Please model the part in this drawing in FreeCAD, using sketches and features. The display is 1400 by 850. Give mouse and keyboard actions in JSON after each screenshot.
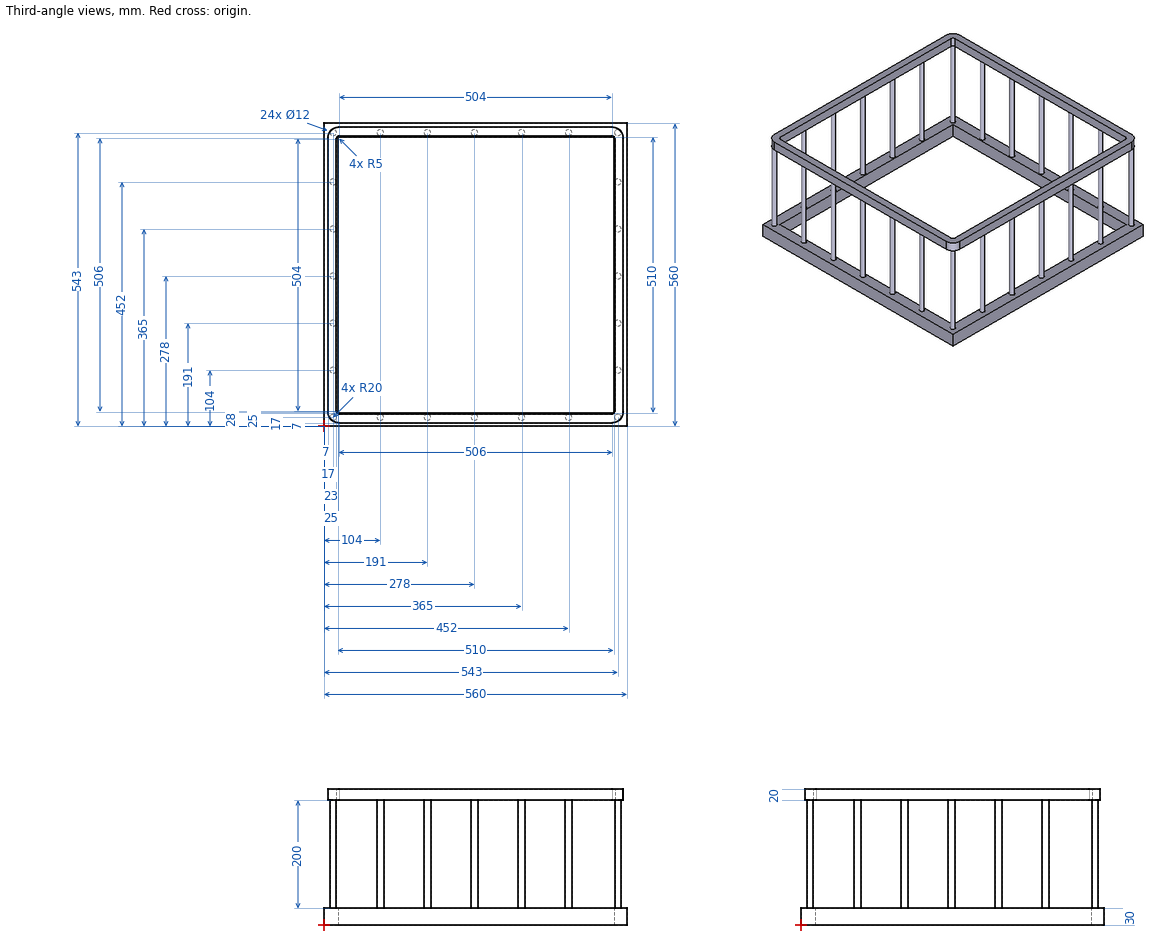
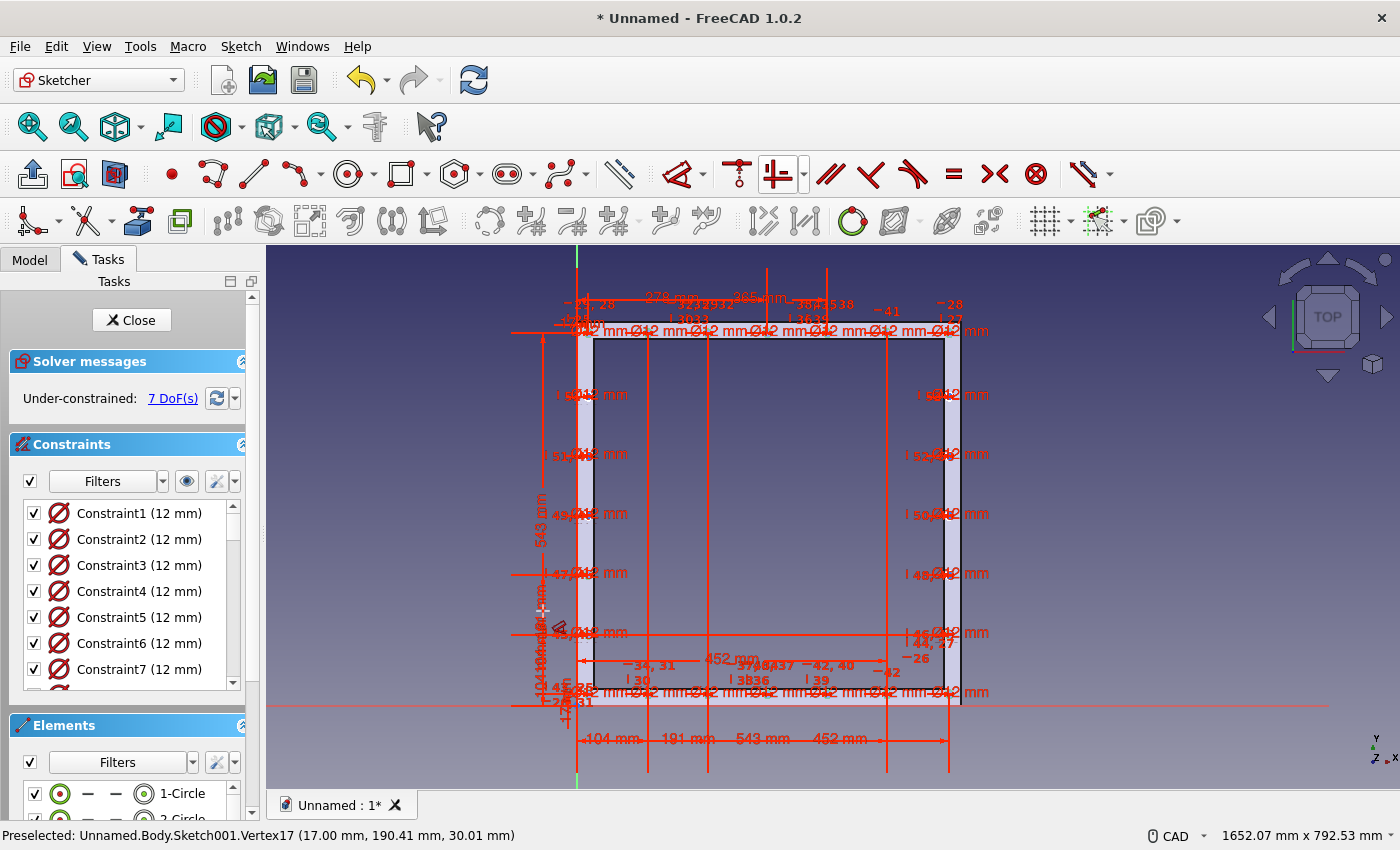
{"action": "left_click", "coordinate": [949, 575]}
{"action": "left_click", "coordinate": [983, 641]}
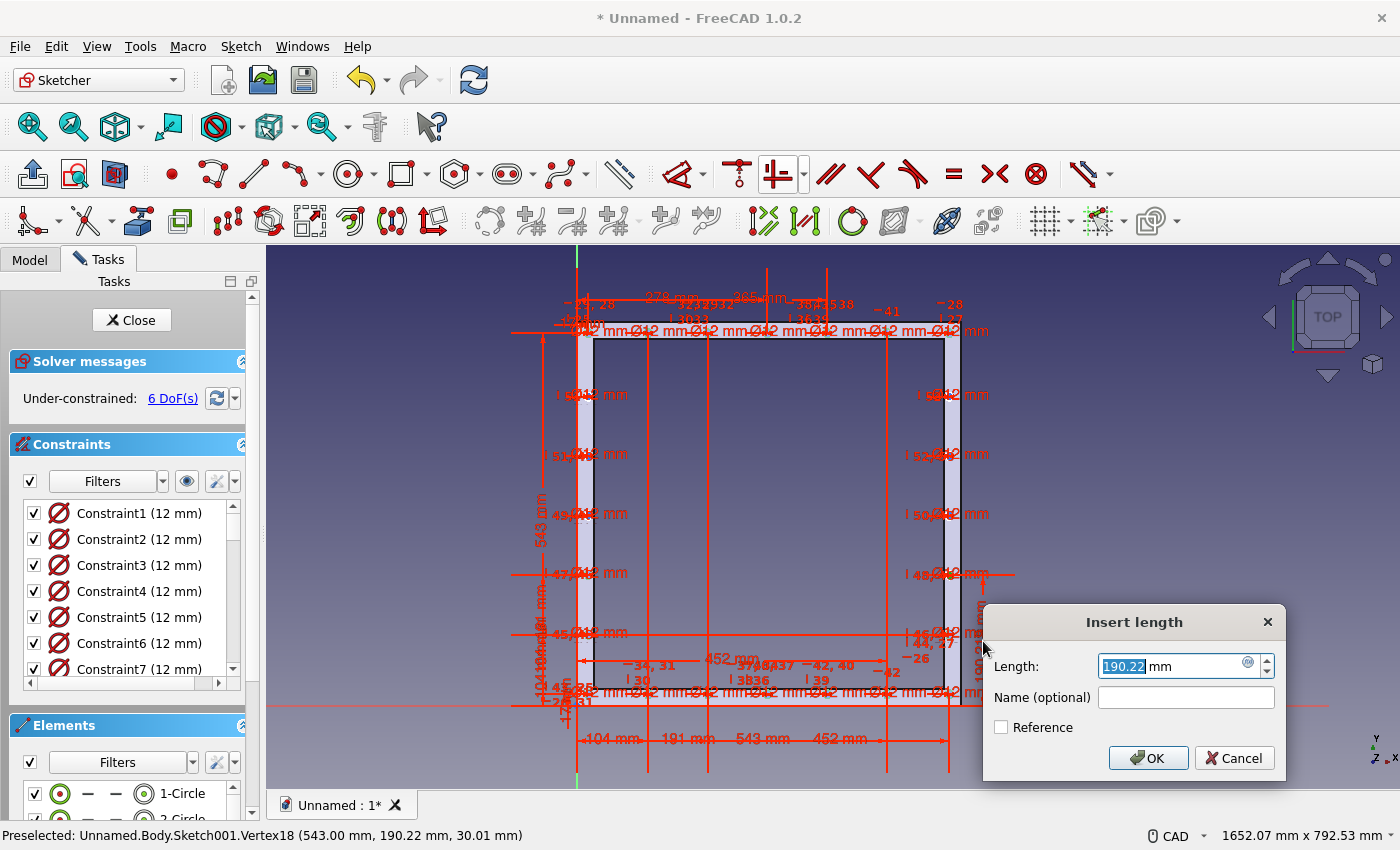
{"action": "type", "text": "191"}
{"action": "key", "text": "Return"}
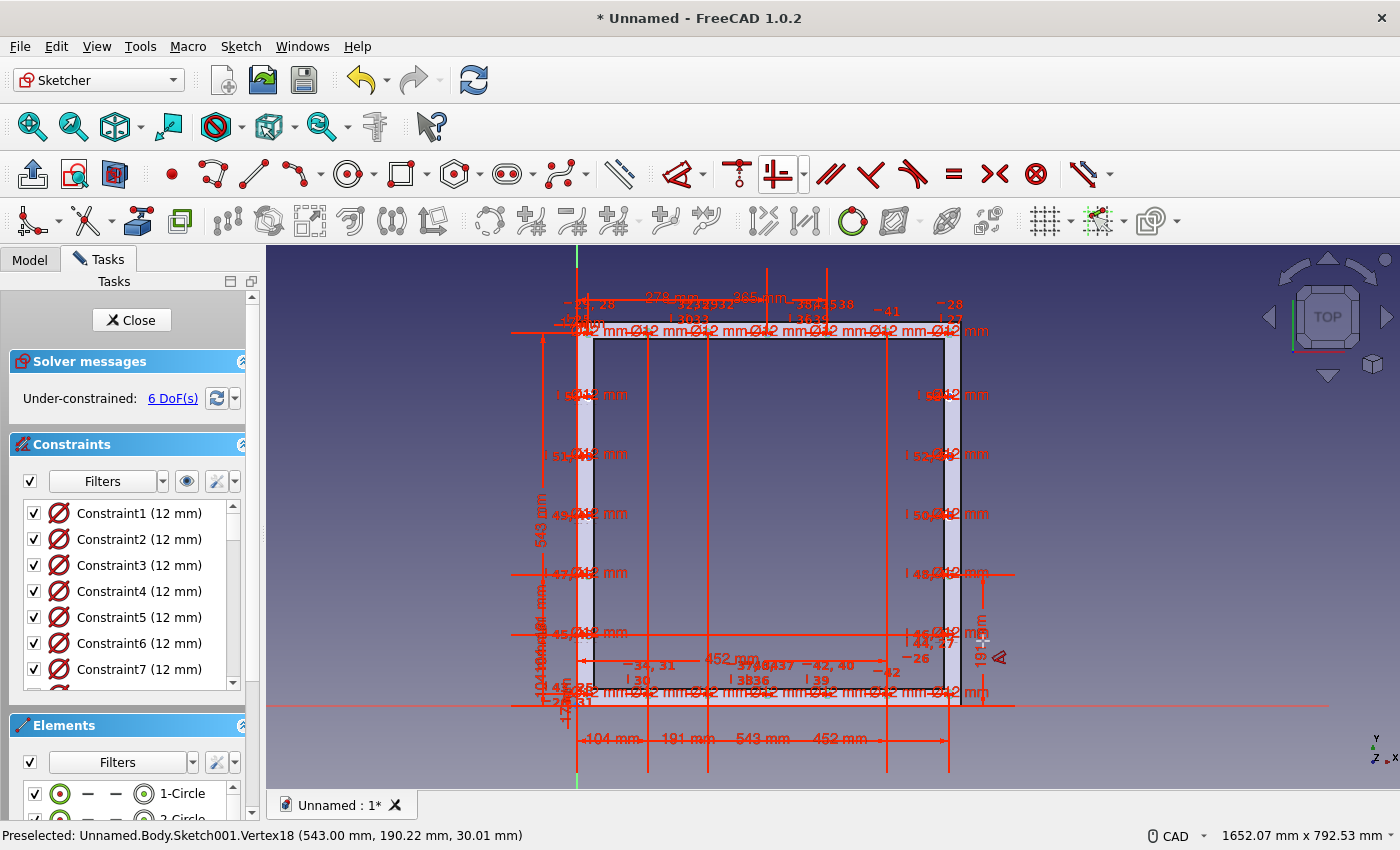
{"action": "left_click", "coordinate": [588, 516]}
{"action": "left_click", "coordinate": [543, 567]}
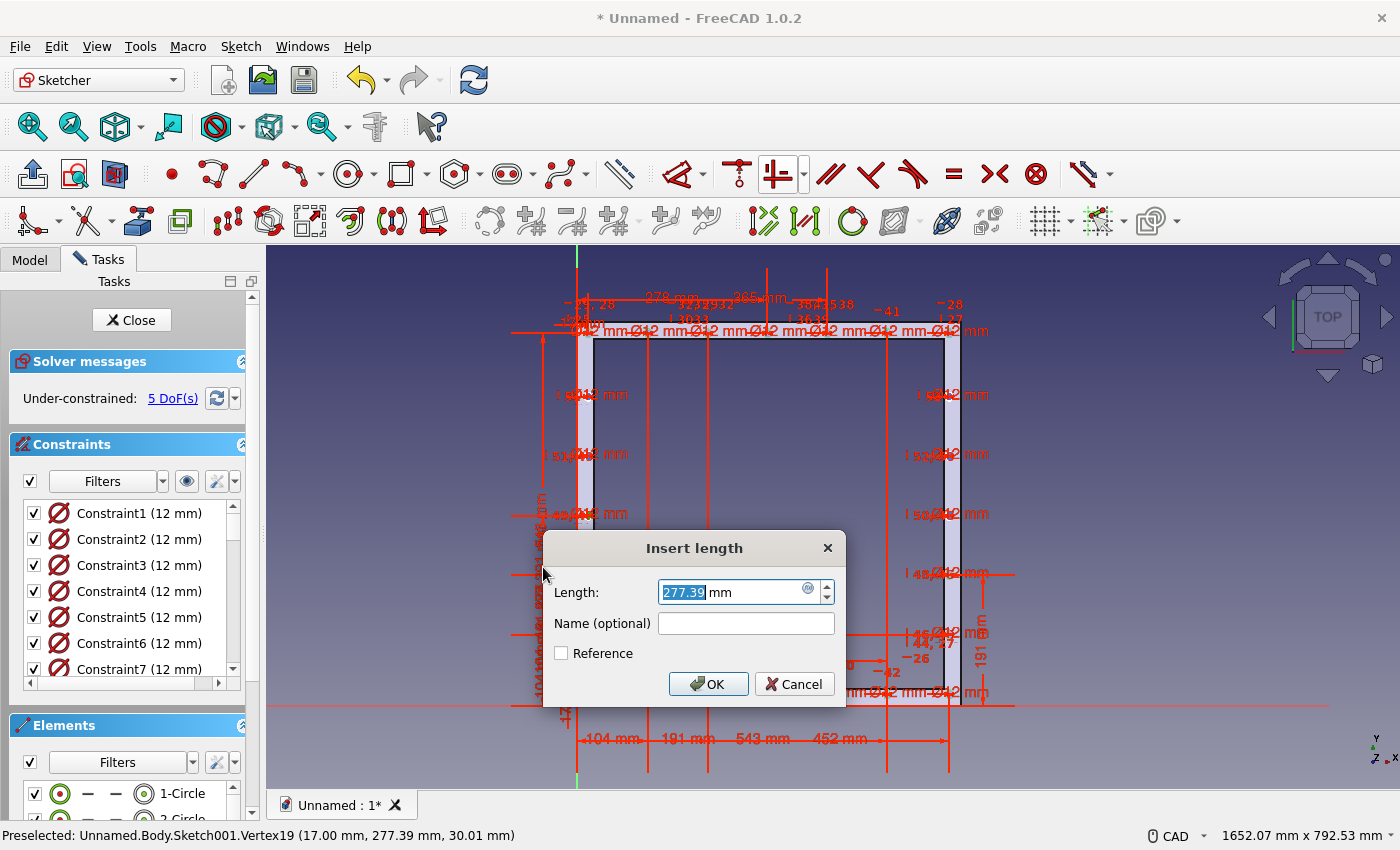
{"action": "type", "text": "278"}
{"action": "key", "text": "Return"}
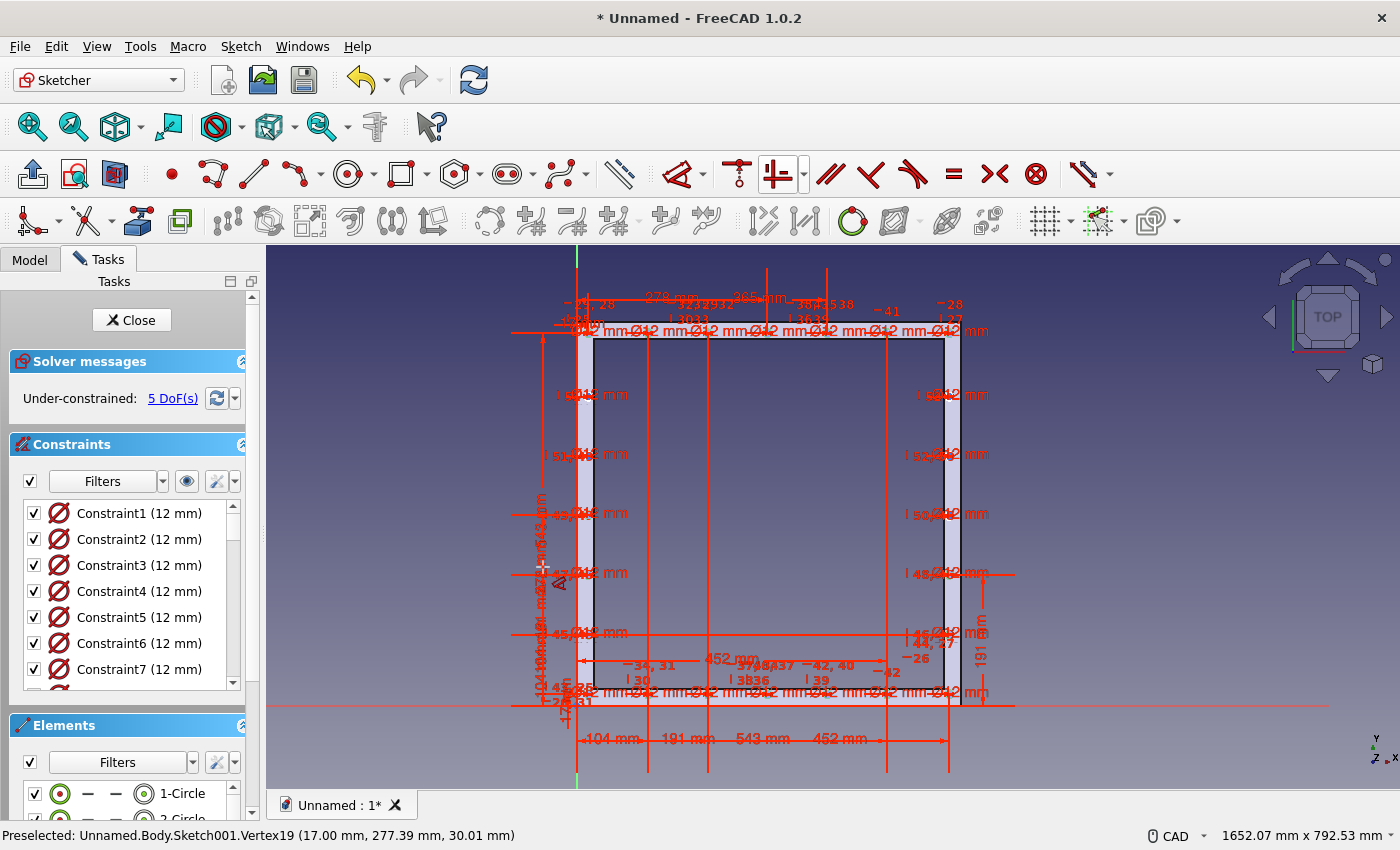
{"action": "left_click", "coordinate": [949, 516]}
{"action": "left_click", "coordinate": [543, 544]}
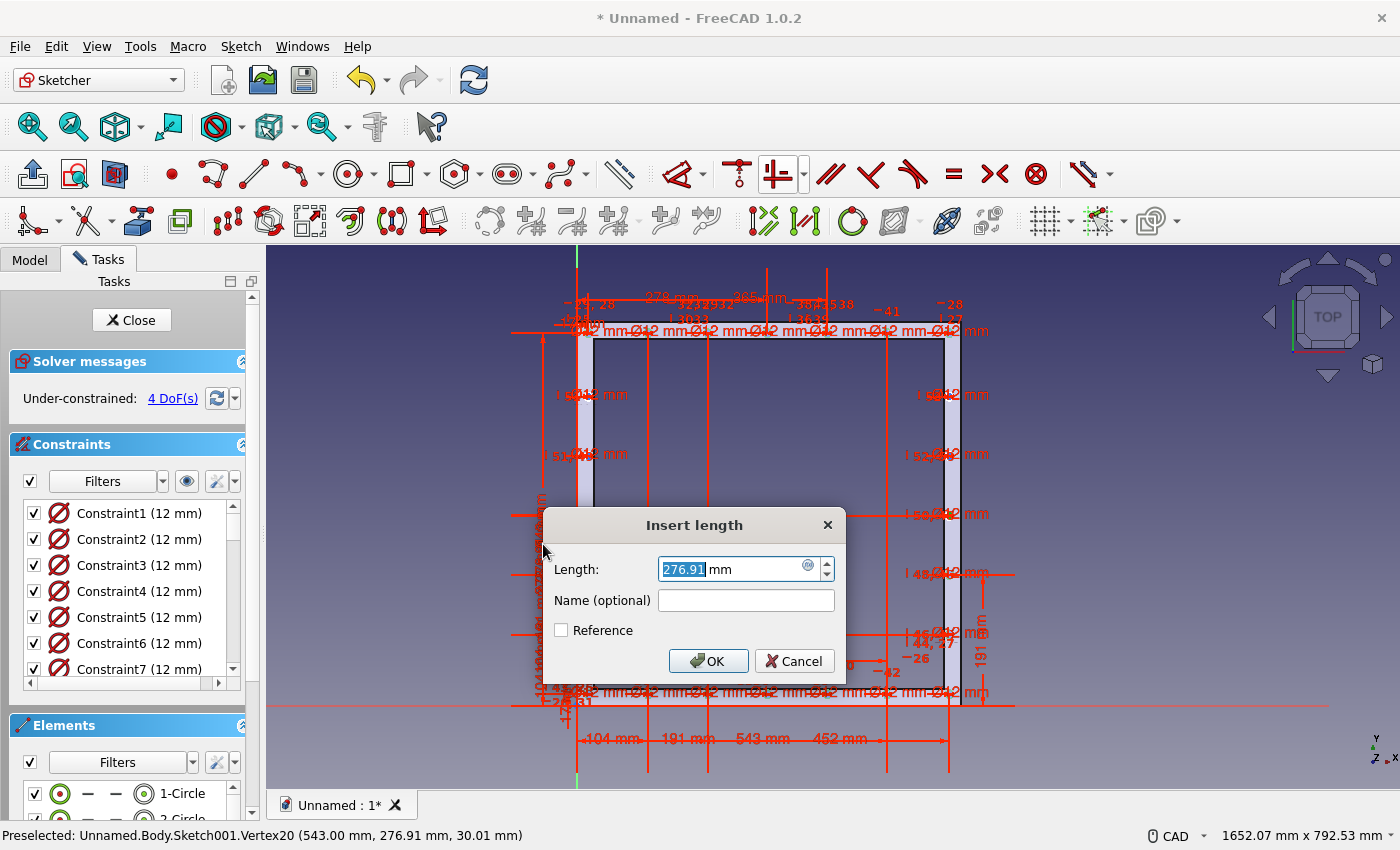
{"action": "type", "text": "278"}
{"action": "key", "text": "Return"}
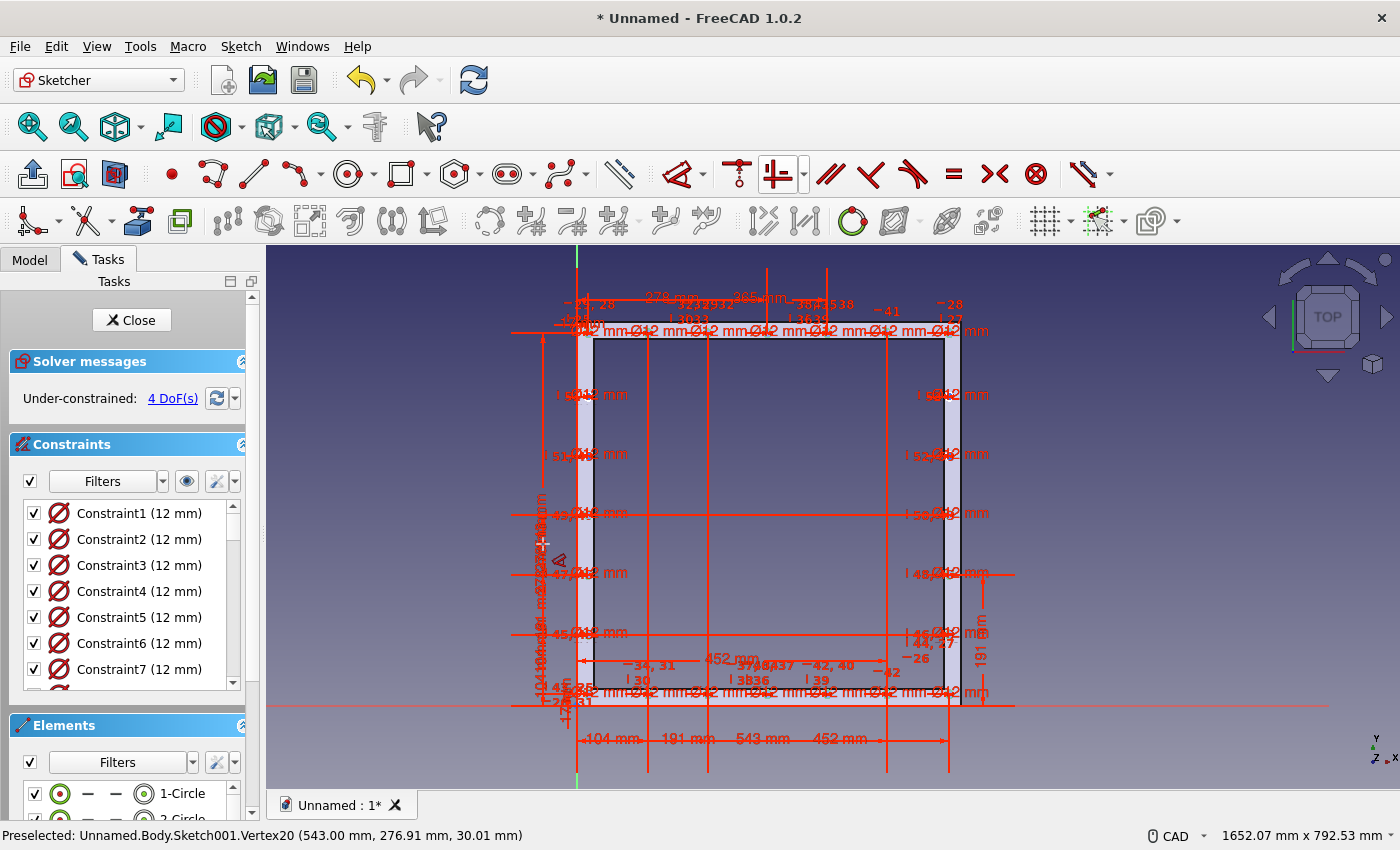
{"action": "left_click", "coordinate": [588, 456]}
{"action": "left_click", "coordinate": [543, 494]}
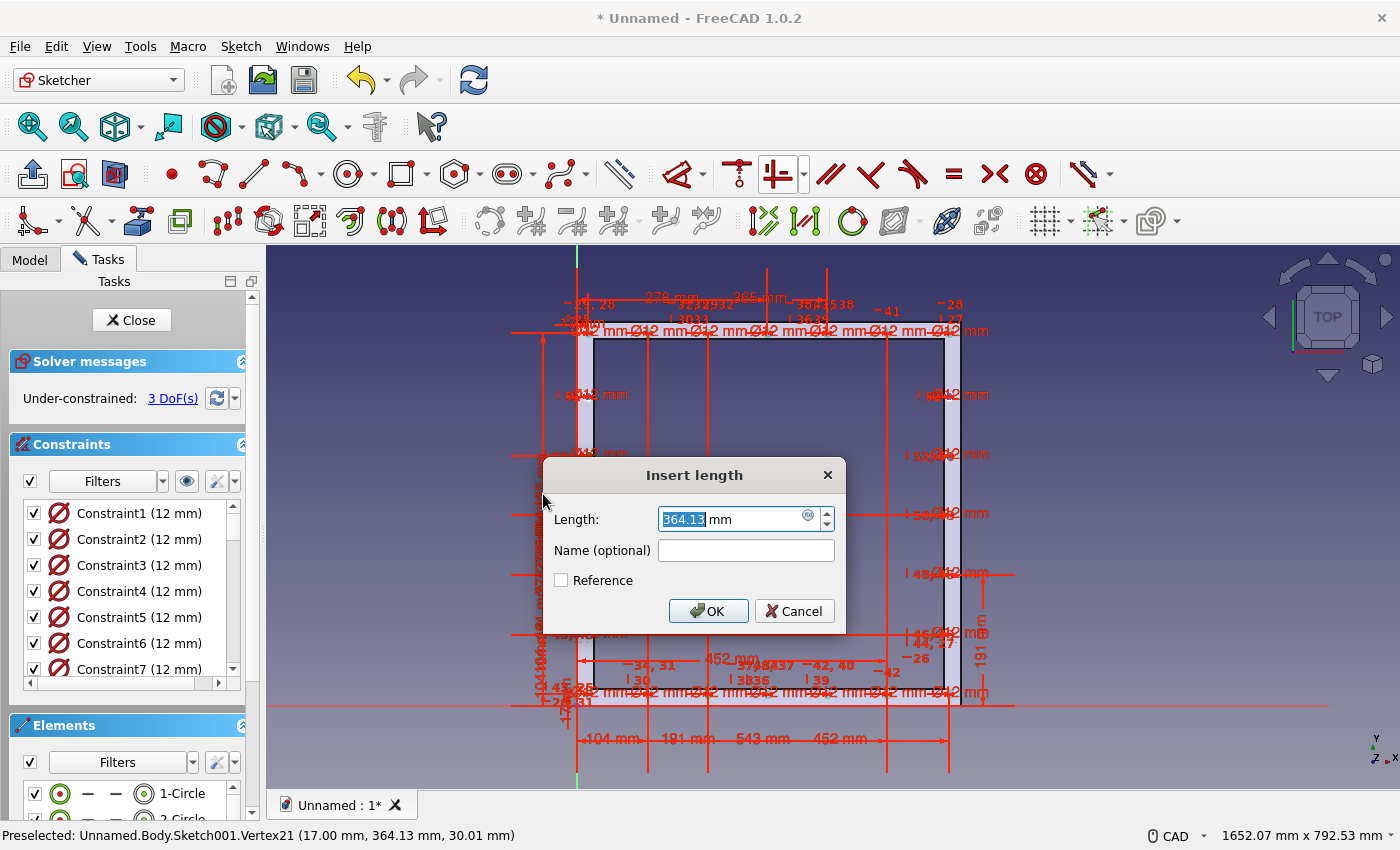
{"action": "type", "text": "365"}
{"action": "key", "text": "Return"}